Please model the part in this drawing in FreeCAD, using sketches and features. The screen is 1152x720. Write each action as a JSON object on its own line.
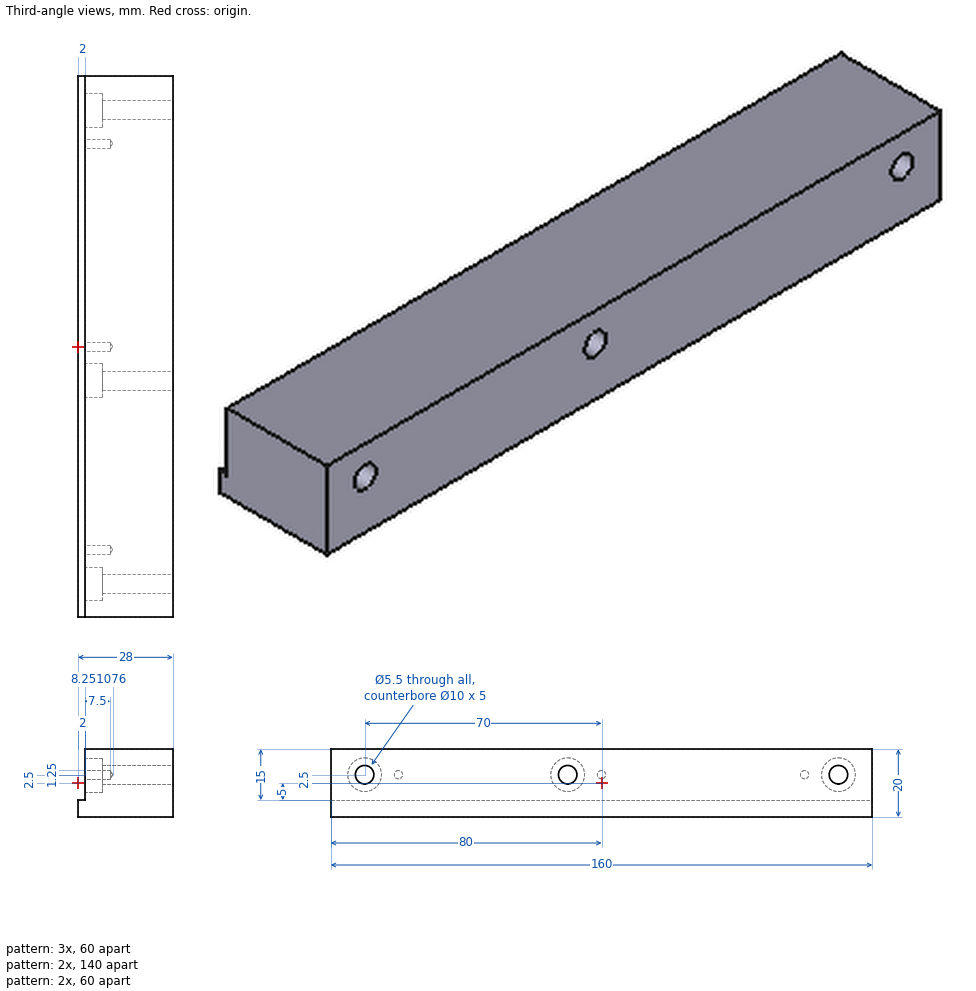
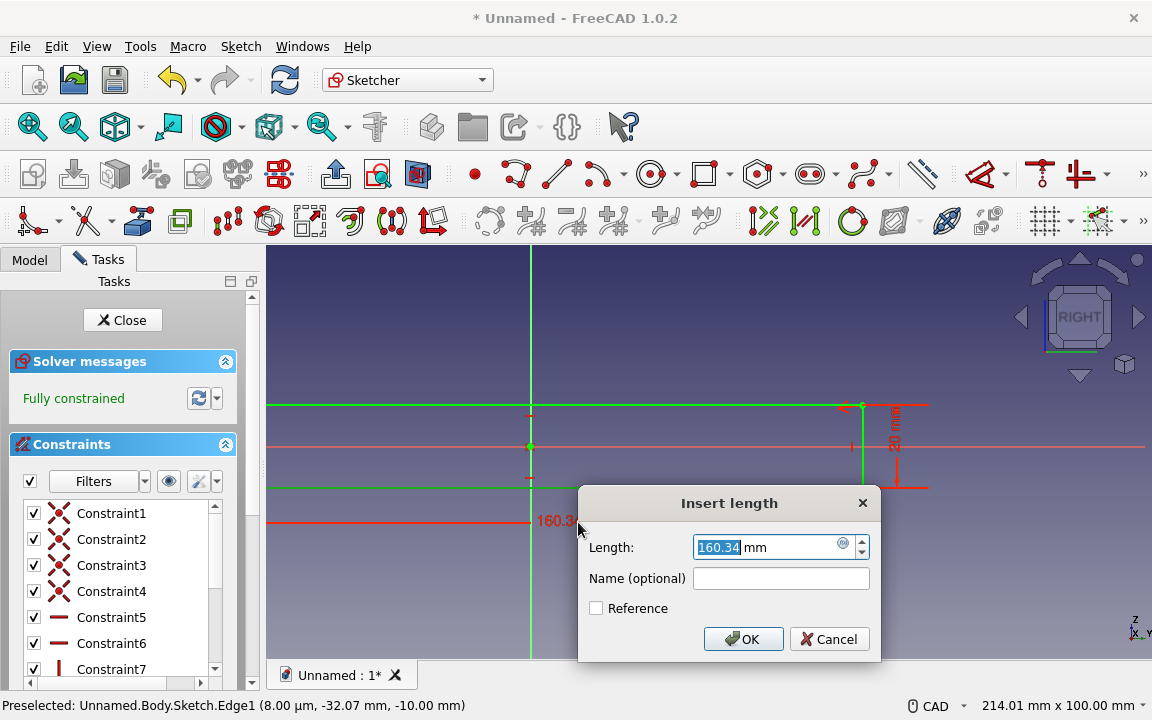
{"action": "type", "text": "160"}
{"action": "key", "text": "Return"}
{"action": "key", "text": "Escape"}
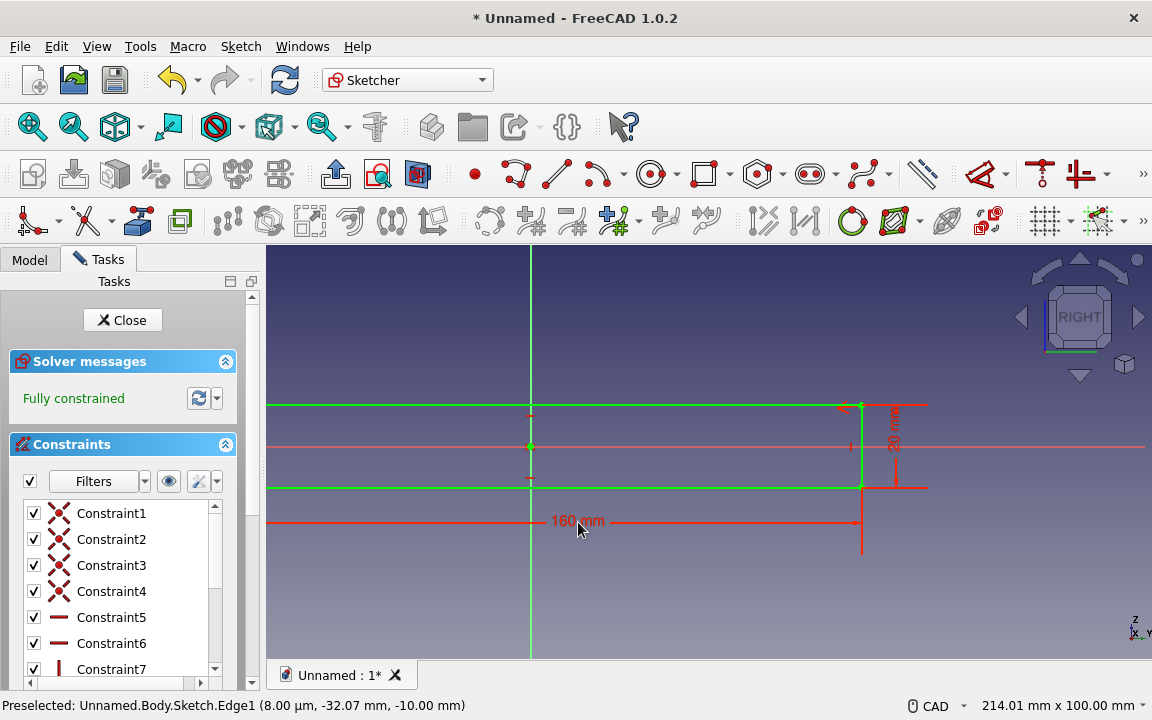
{"action": "left_click", "coordinate": [123, 320]}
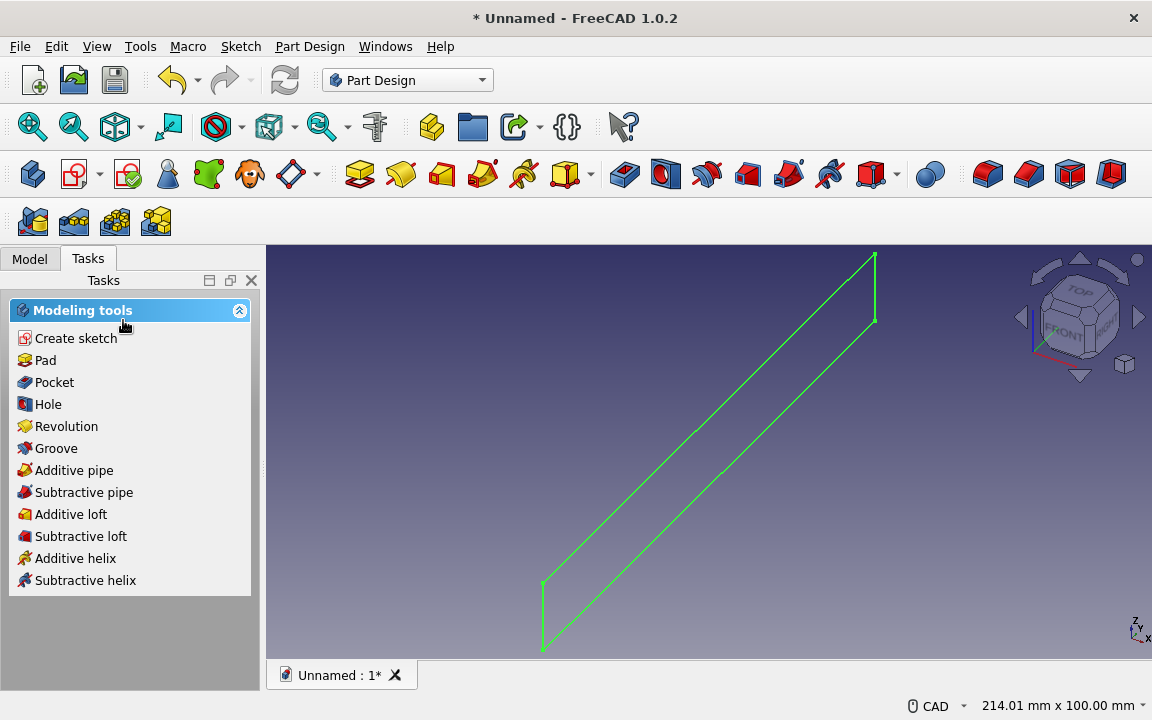
{"action": "left_click", "coordinate": [360, 174]}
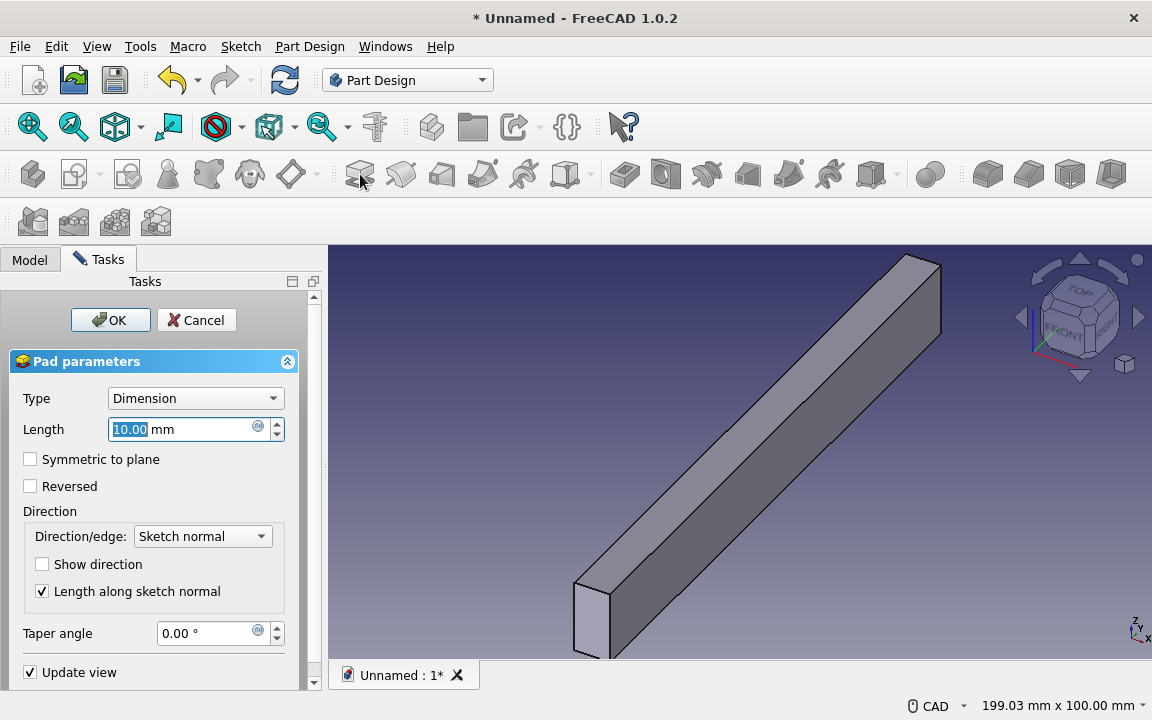
{"action": "type", "text": "28"}
{"action": "key", "text": "Tab"}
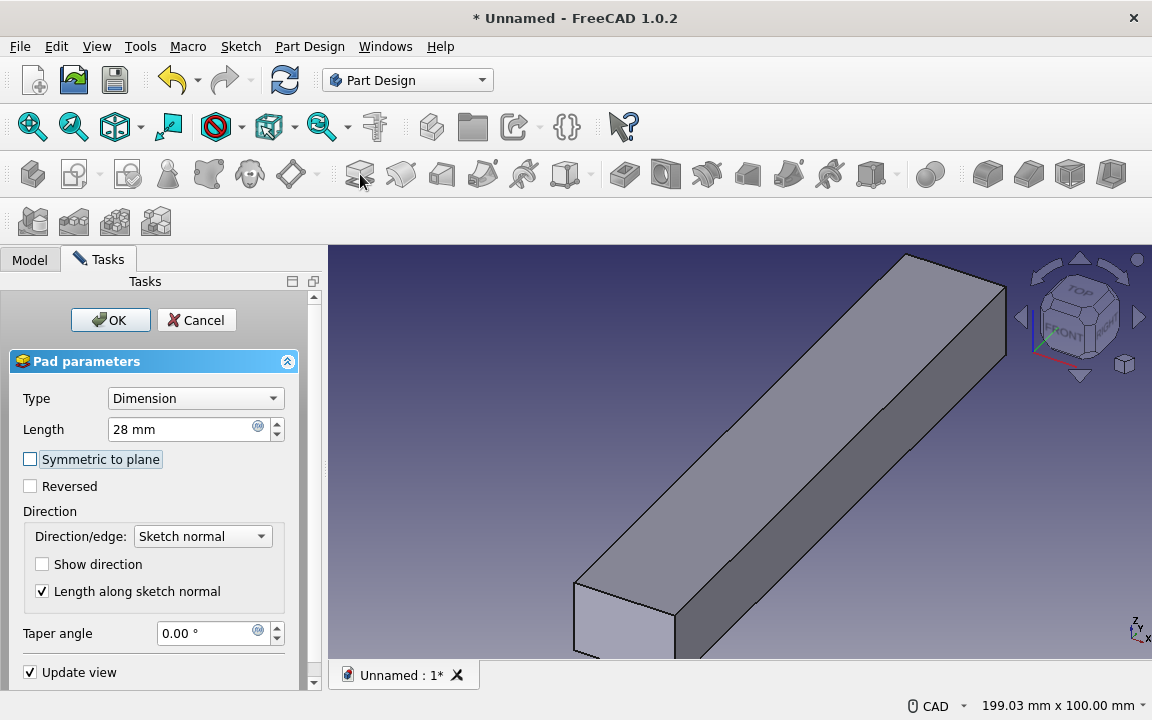
{"action": "left_click", "coordinate": [111, 320]}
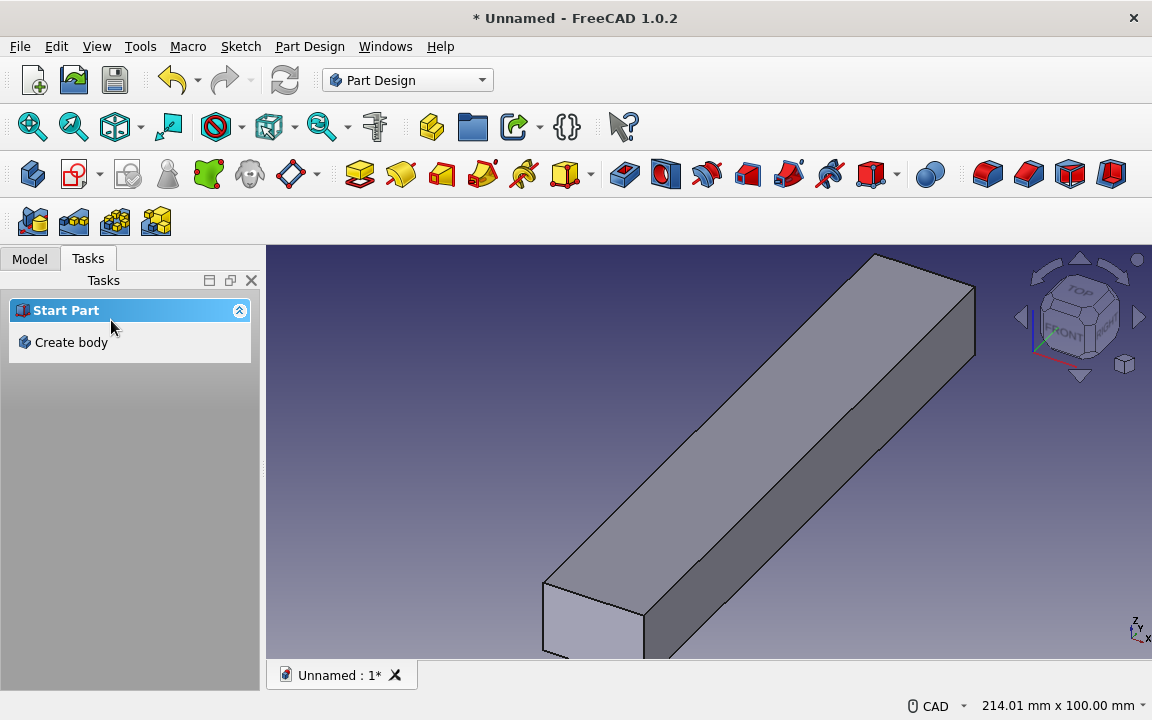
{"action": "key", "text": "v f"}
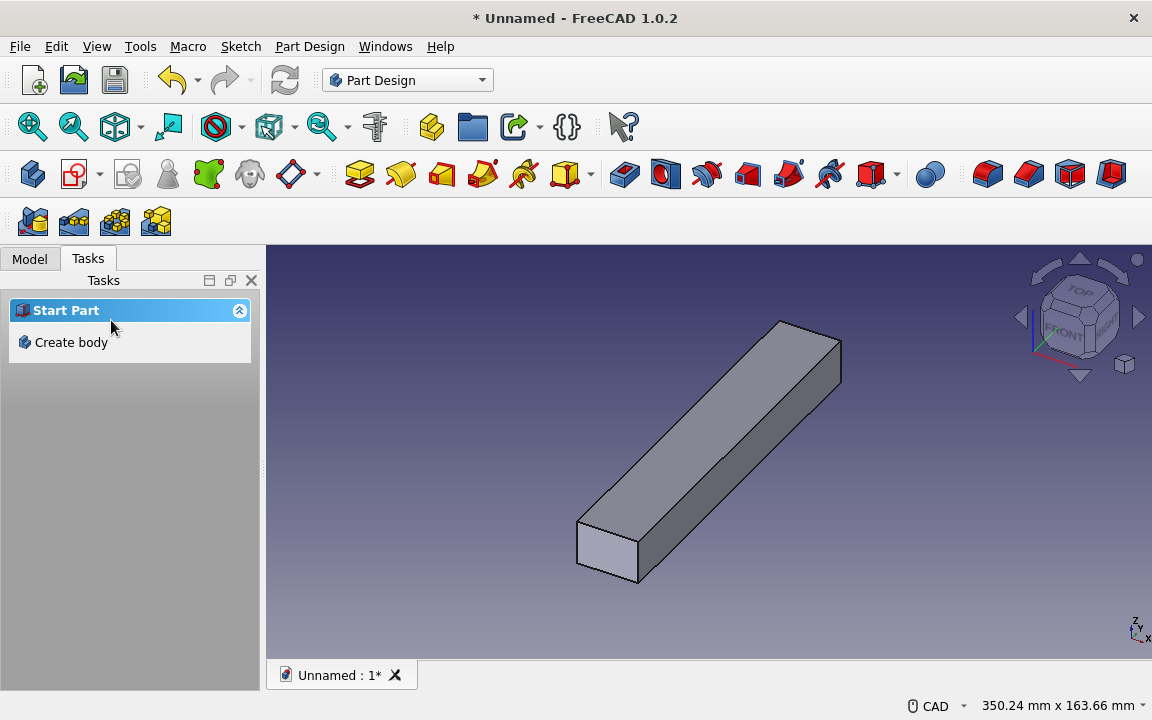
{"action": "key", "text": "6"}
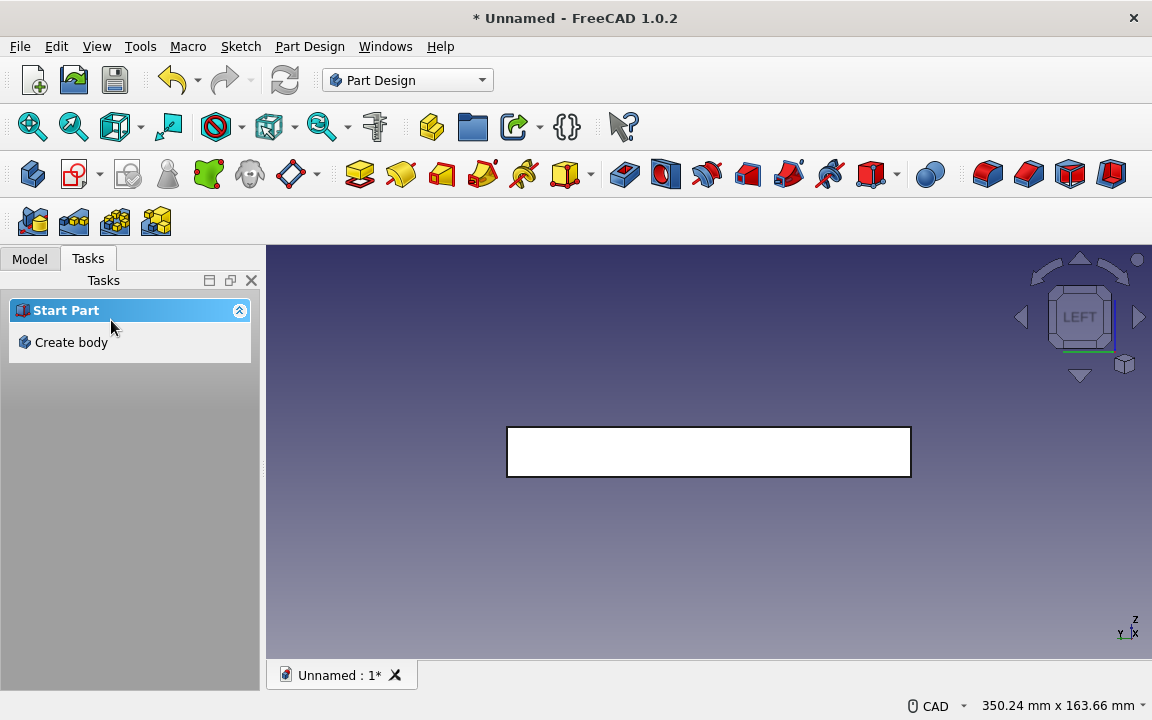
{"action": "left_click", "coordinate": [536, 451]}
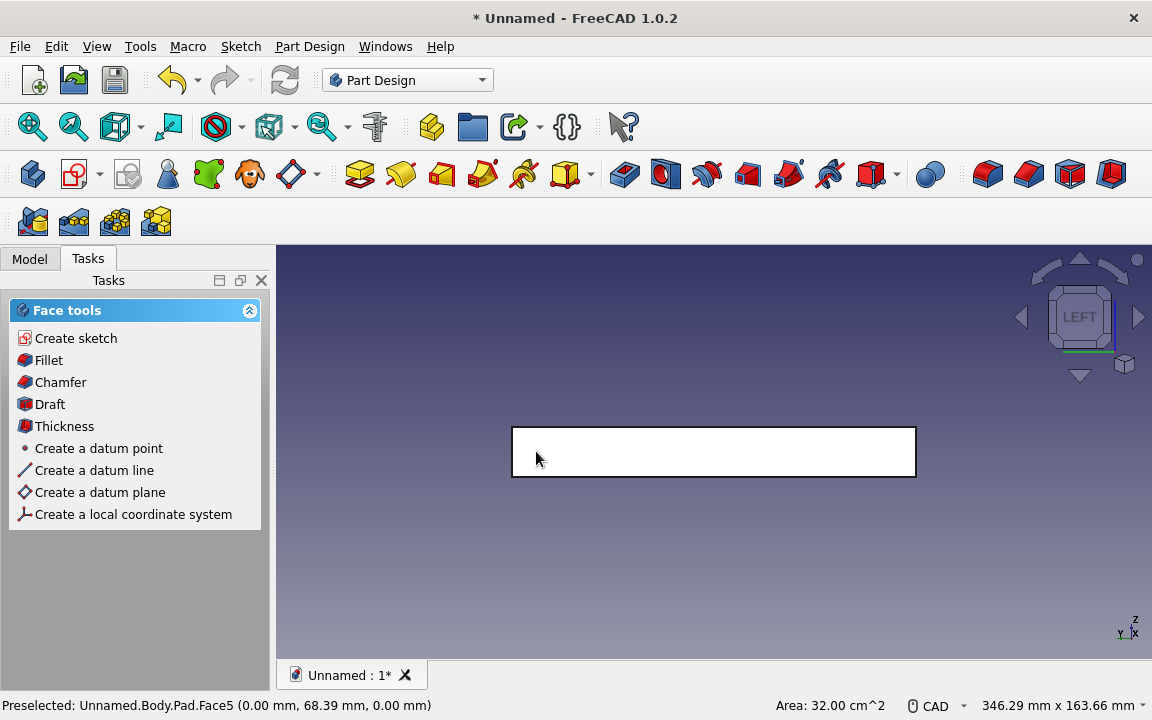
{"action": "left_click", "coordinate": [74, 174]}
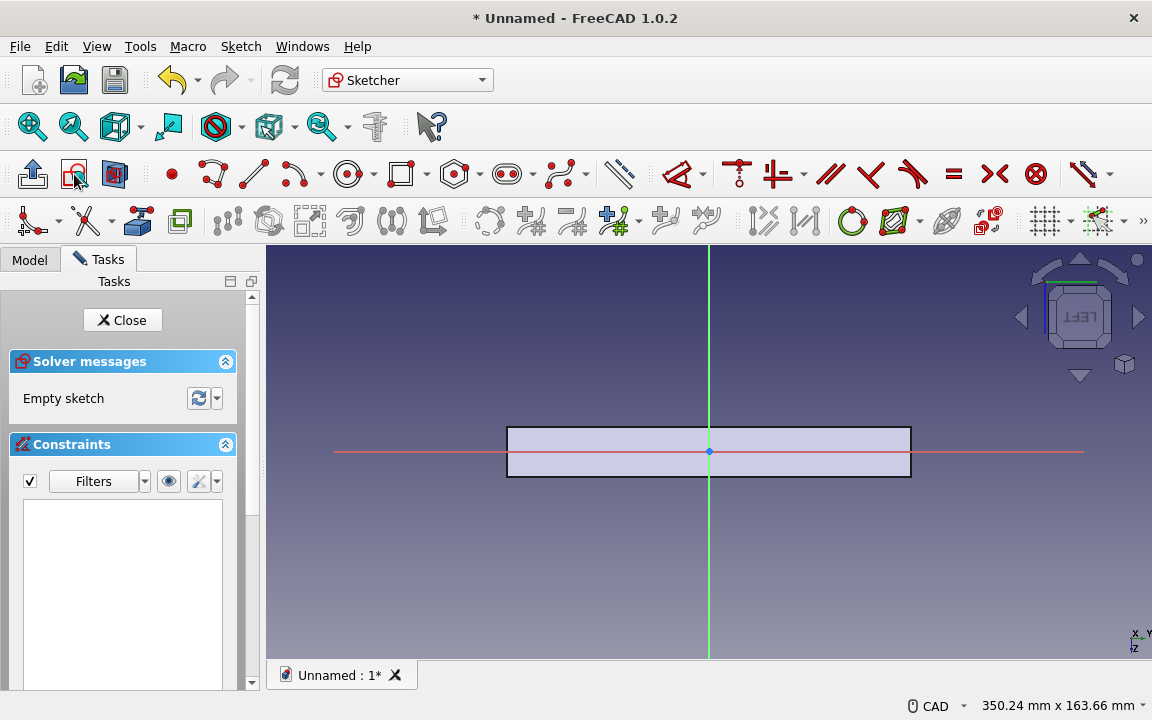
{"action": "key", "text": "g r"}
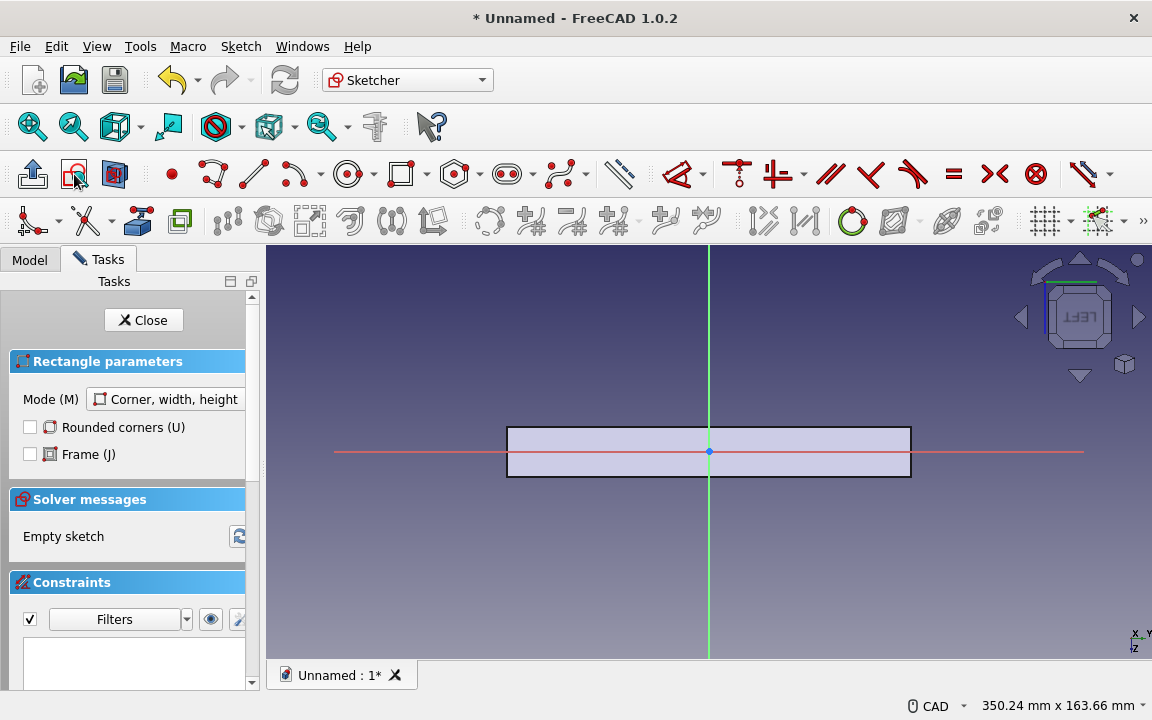
{"action": "scroll", "coordinate": [507, 439], "scroll_direction": "up", "scroll_amount": 2}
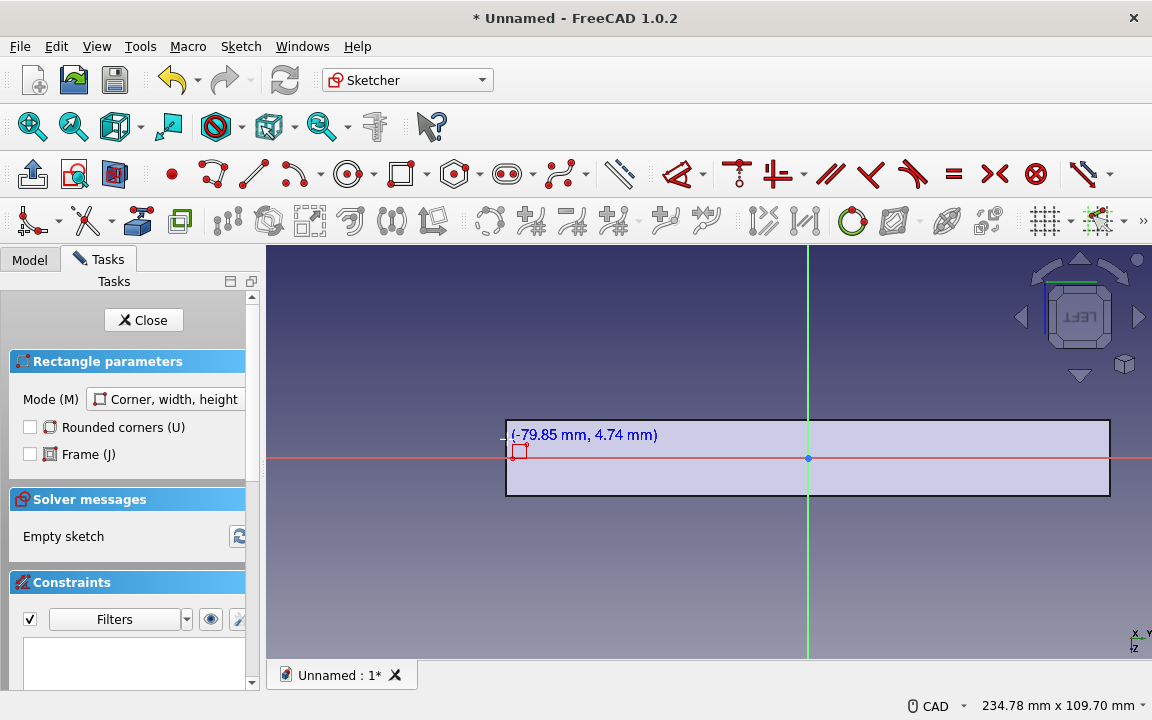
{"action": "left_click", "coordinate": [506, 439]}